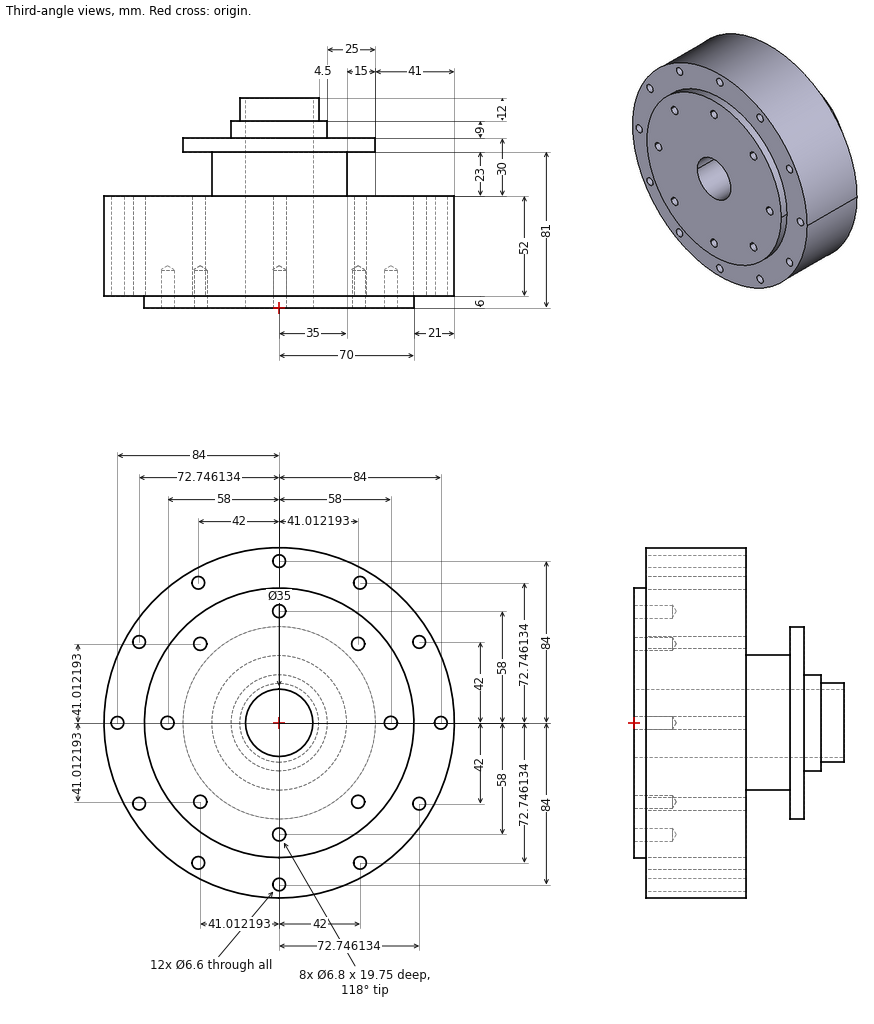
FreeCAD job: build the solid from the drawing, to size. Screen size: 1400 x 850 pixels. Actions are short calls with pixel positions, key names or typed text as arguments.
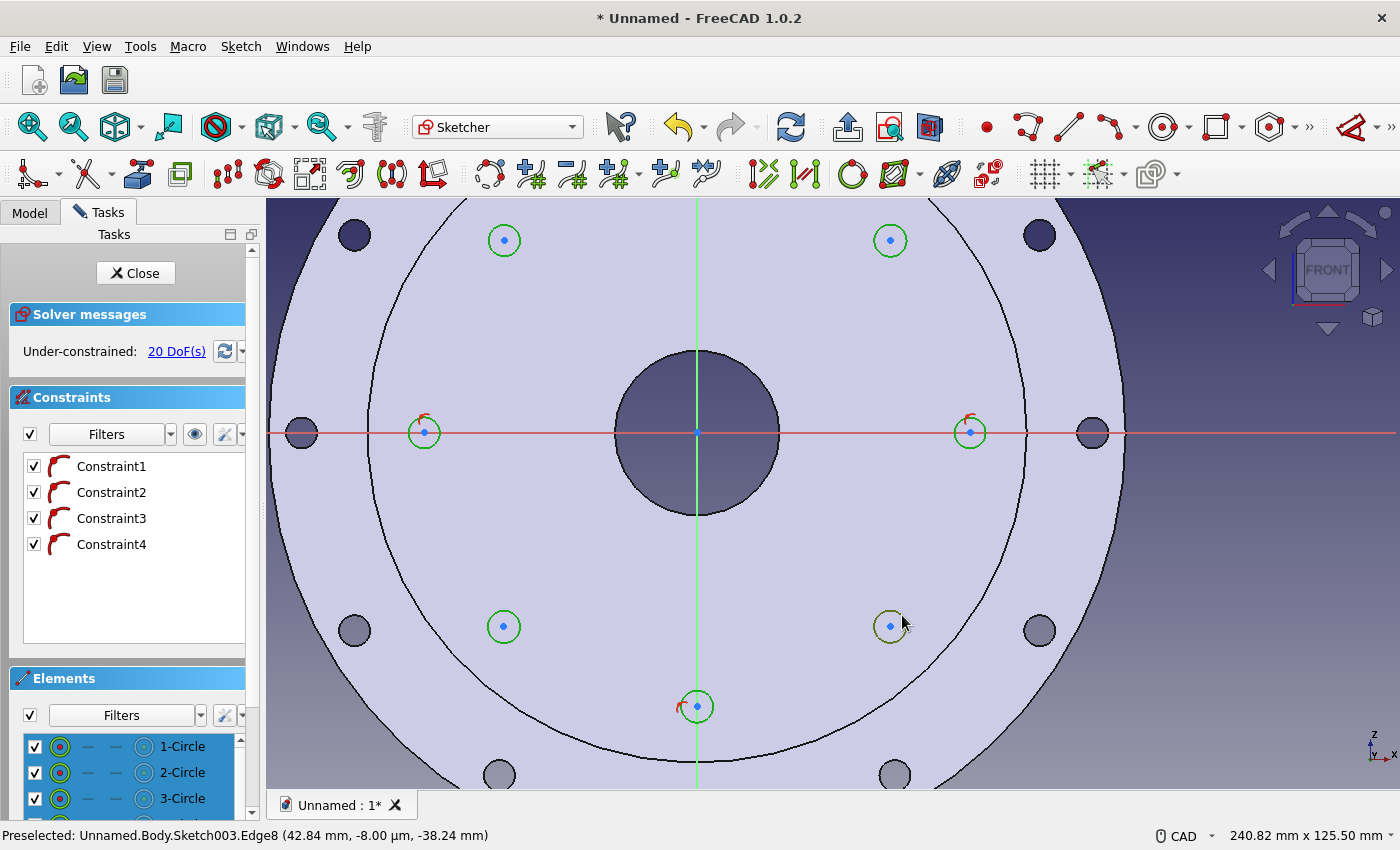
key(e)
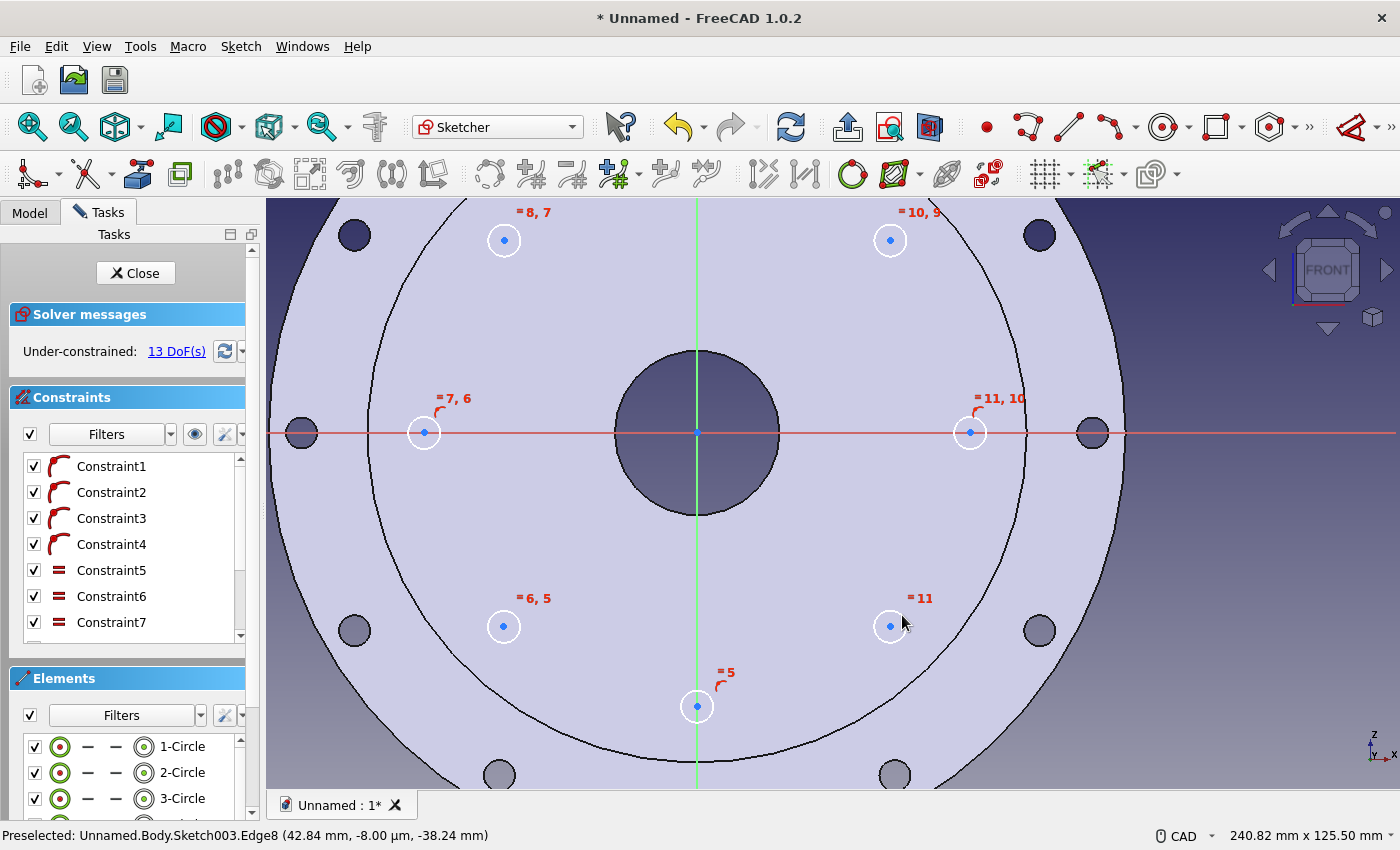
click(1350, 128)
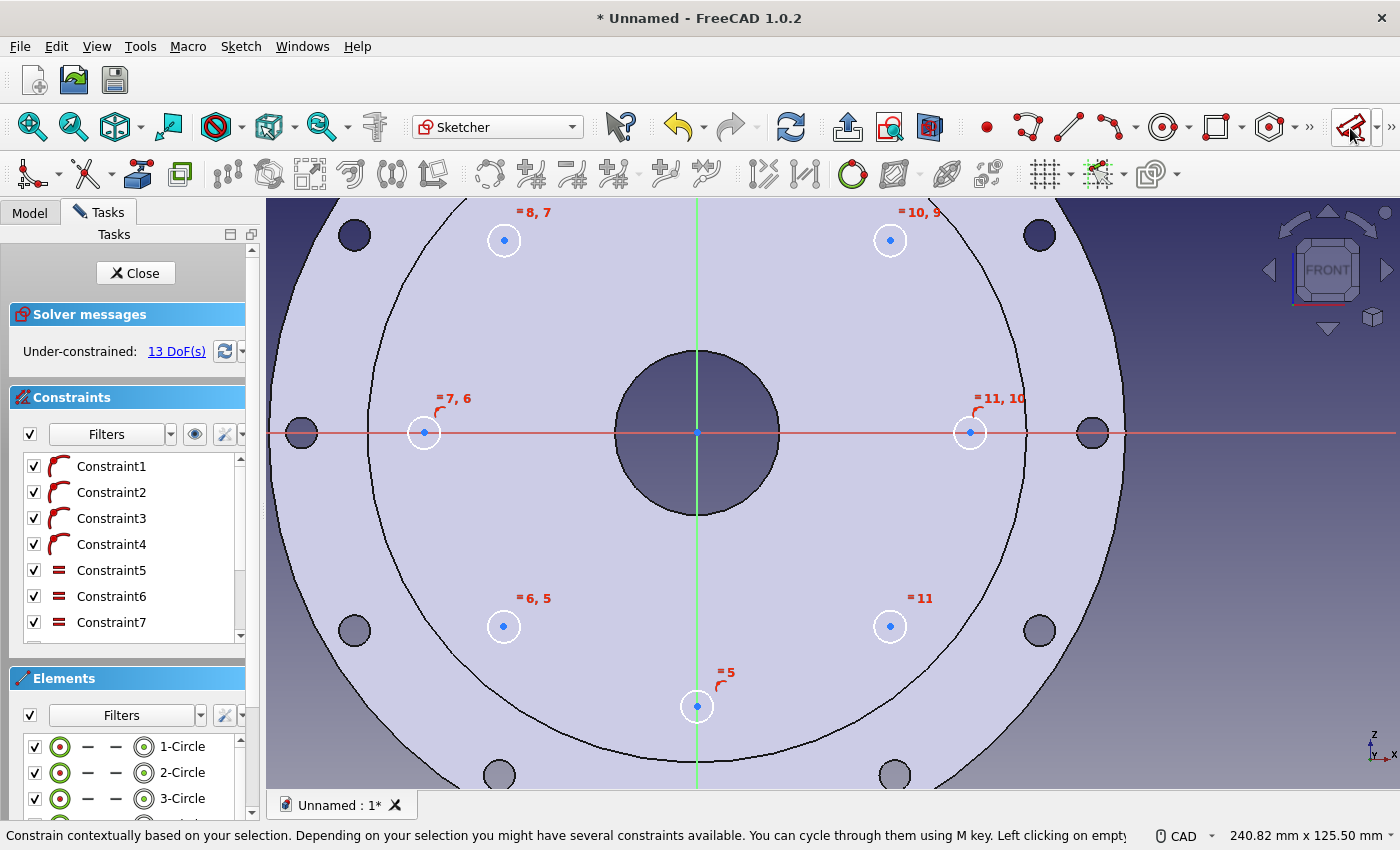
scroll(708, 695, up, 2)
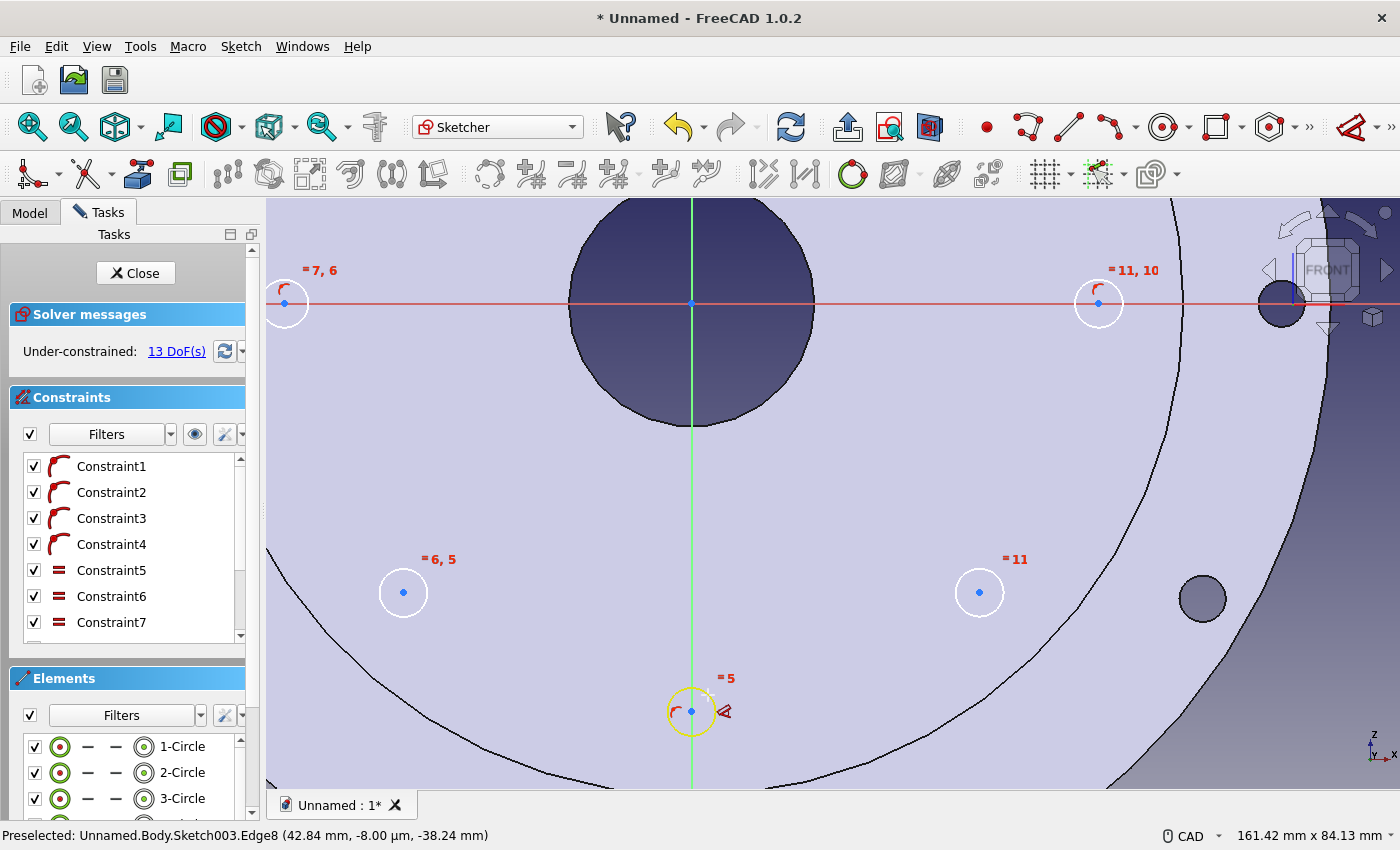
click(708, 695)
click(730, 672)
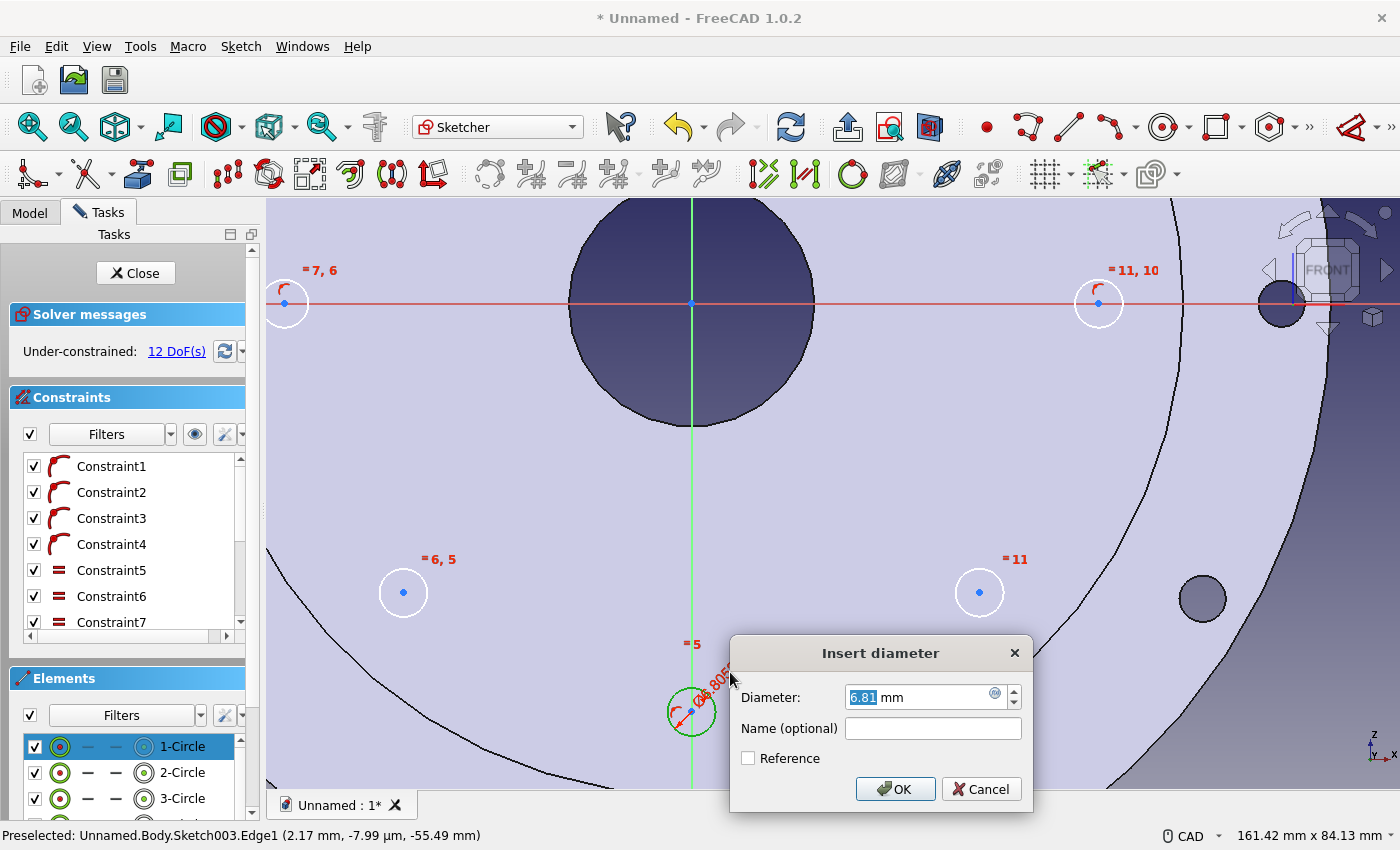
text(6.8)
key(Return)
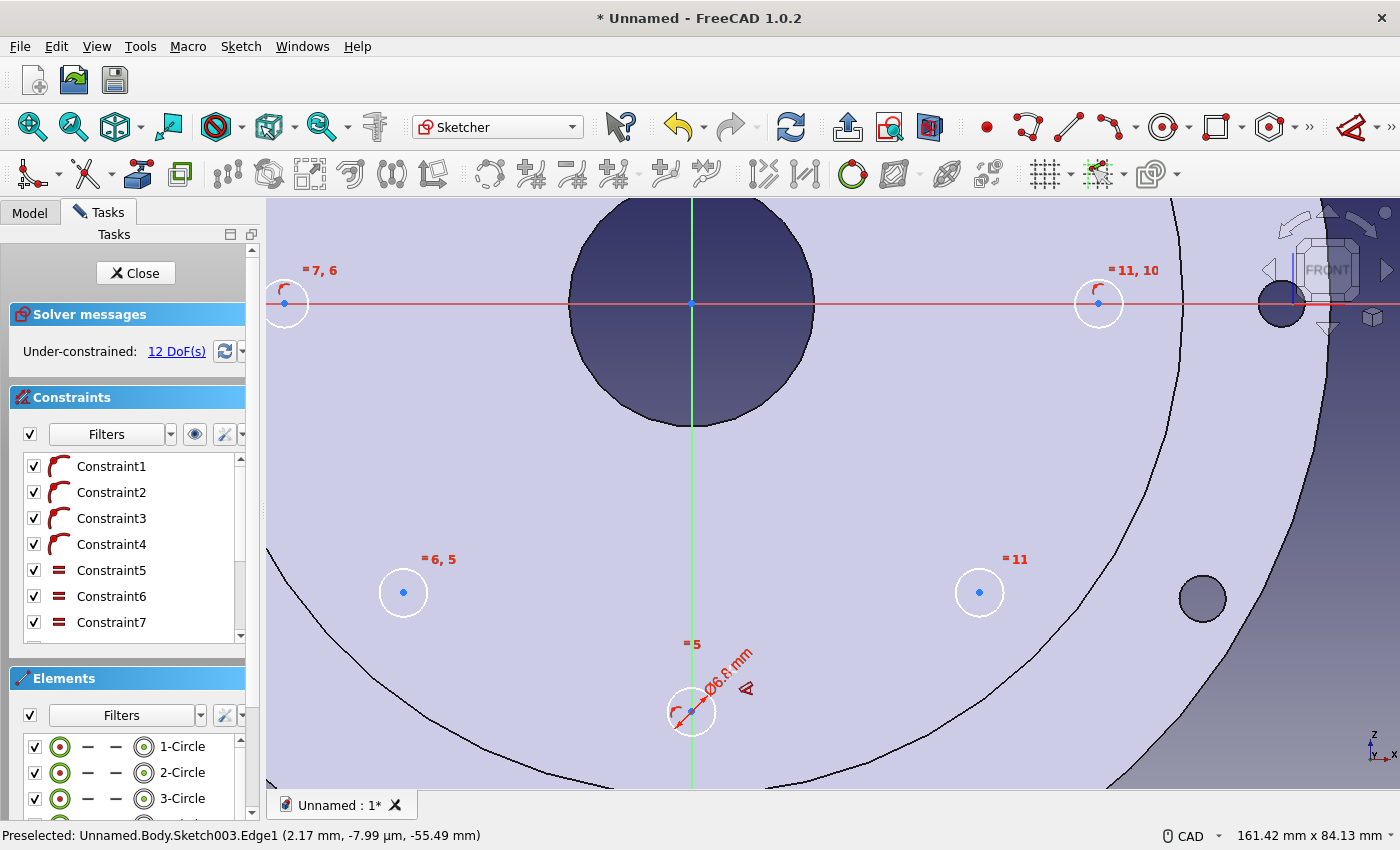
click(692, 712)
click(726, 508)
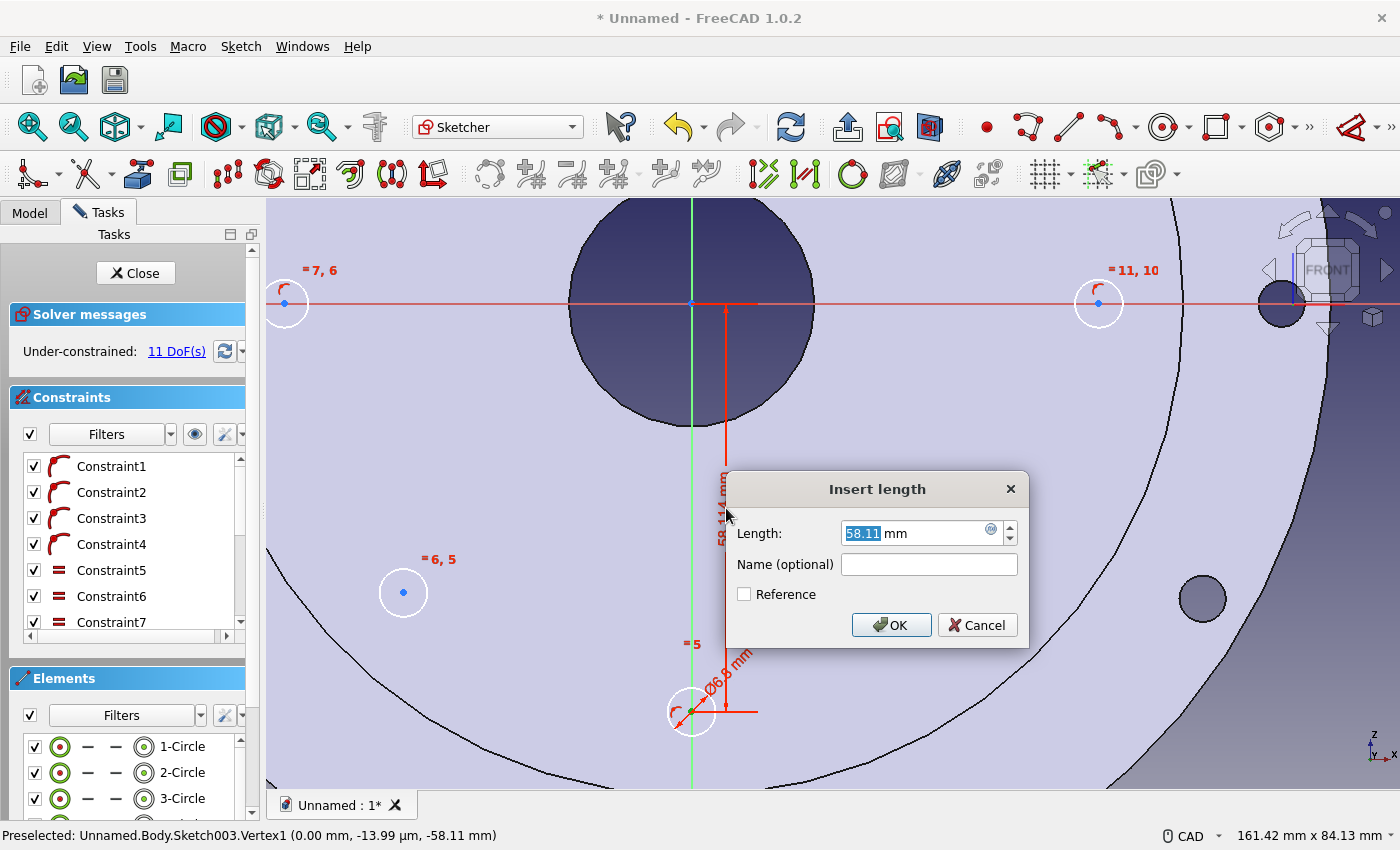
text(58)
key(Return)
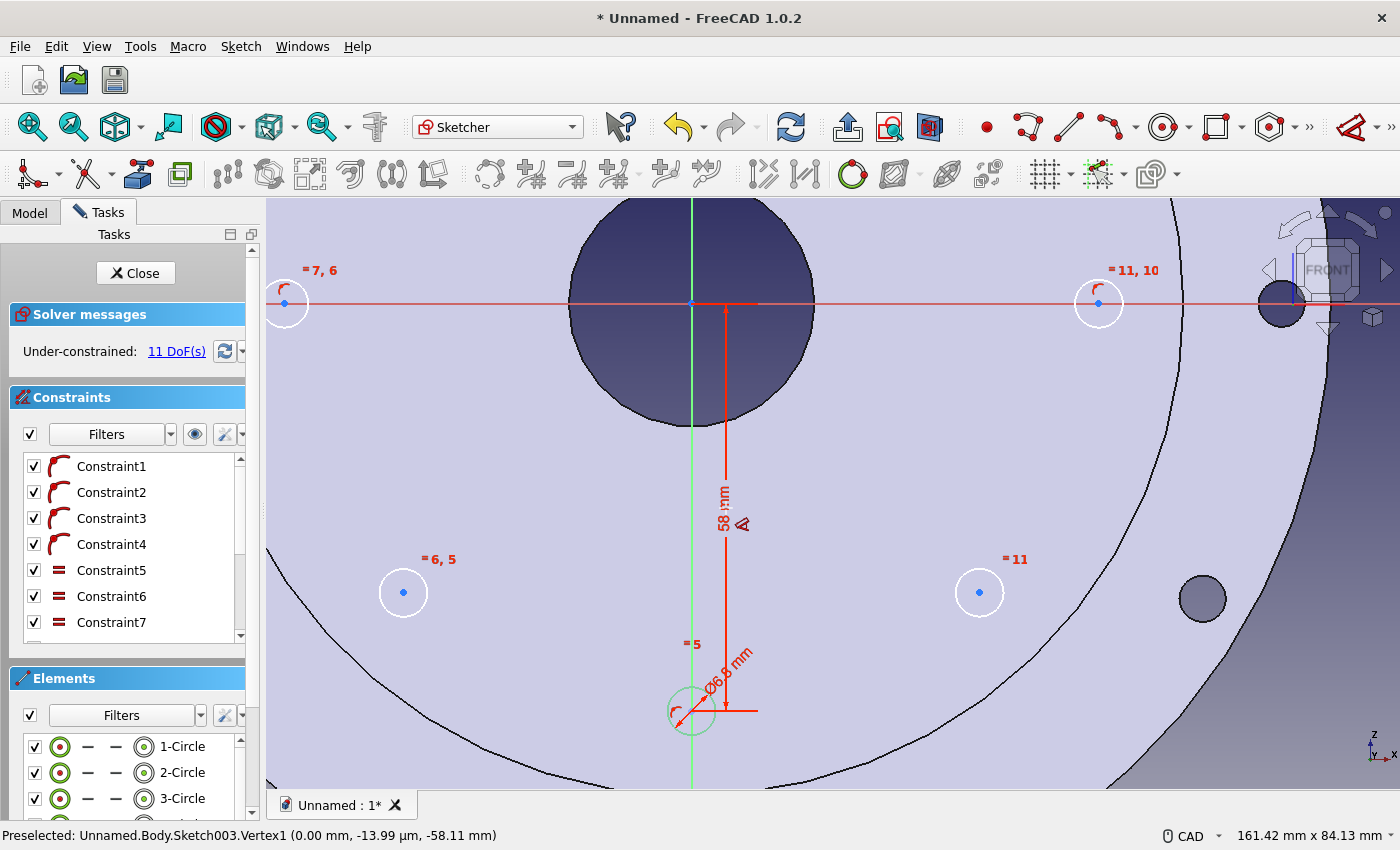
scroll(824, 648, down, 4)